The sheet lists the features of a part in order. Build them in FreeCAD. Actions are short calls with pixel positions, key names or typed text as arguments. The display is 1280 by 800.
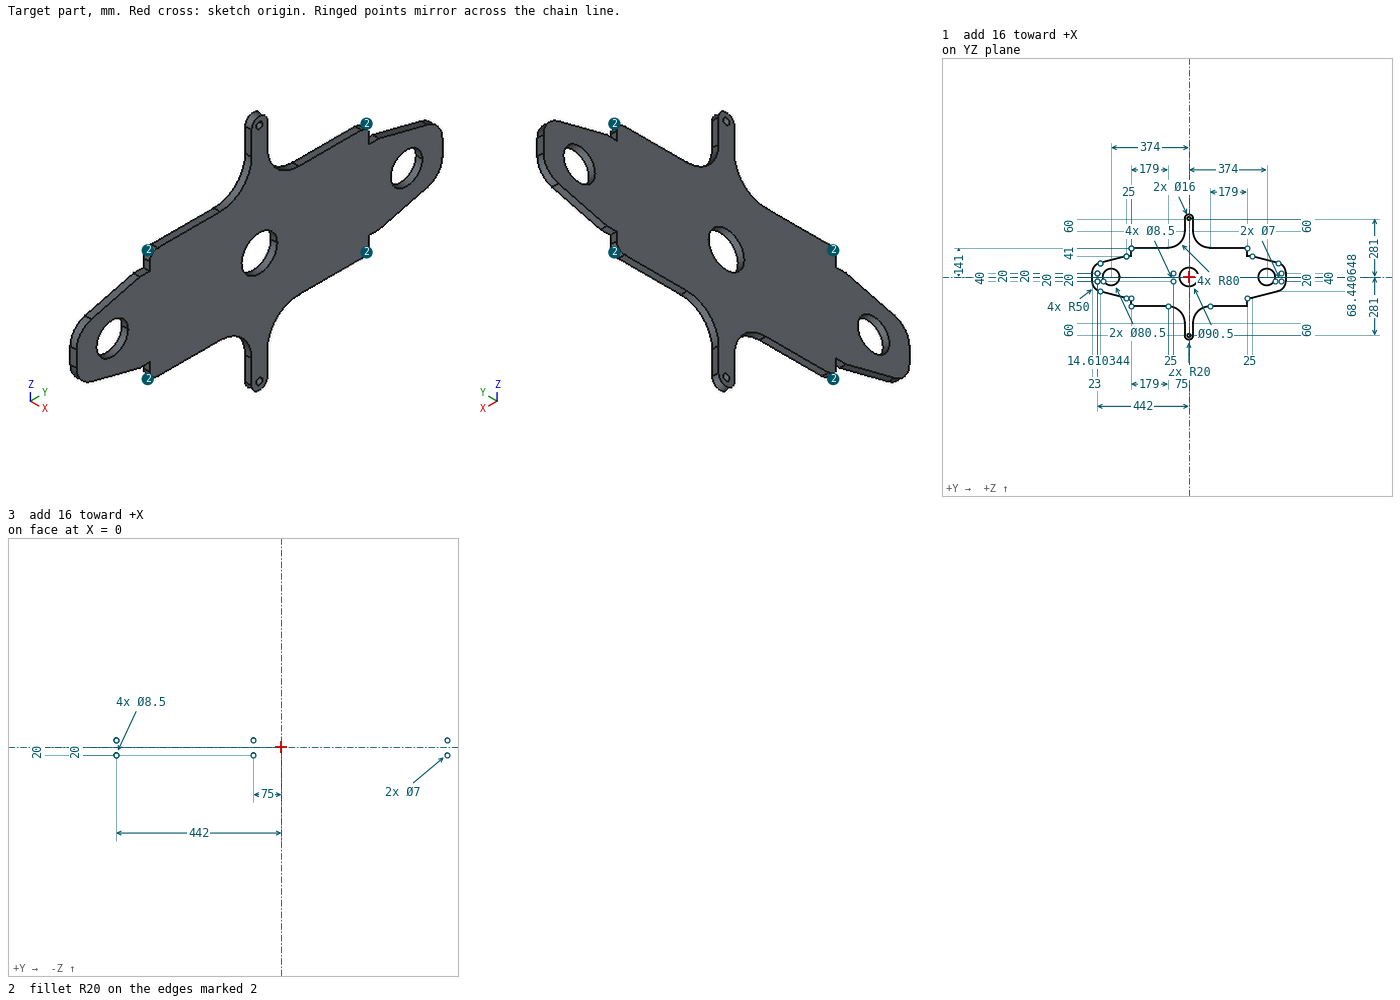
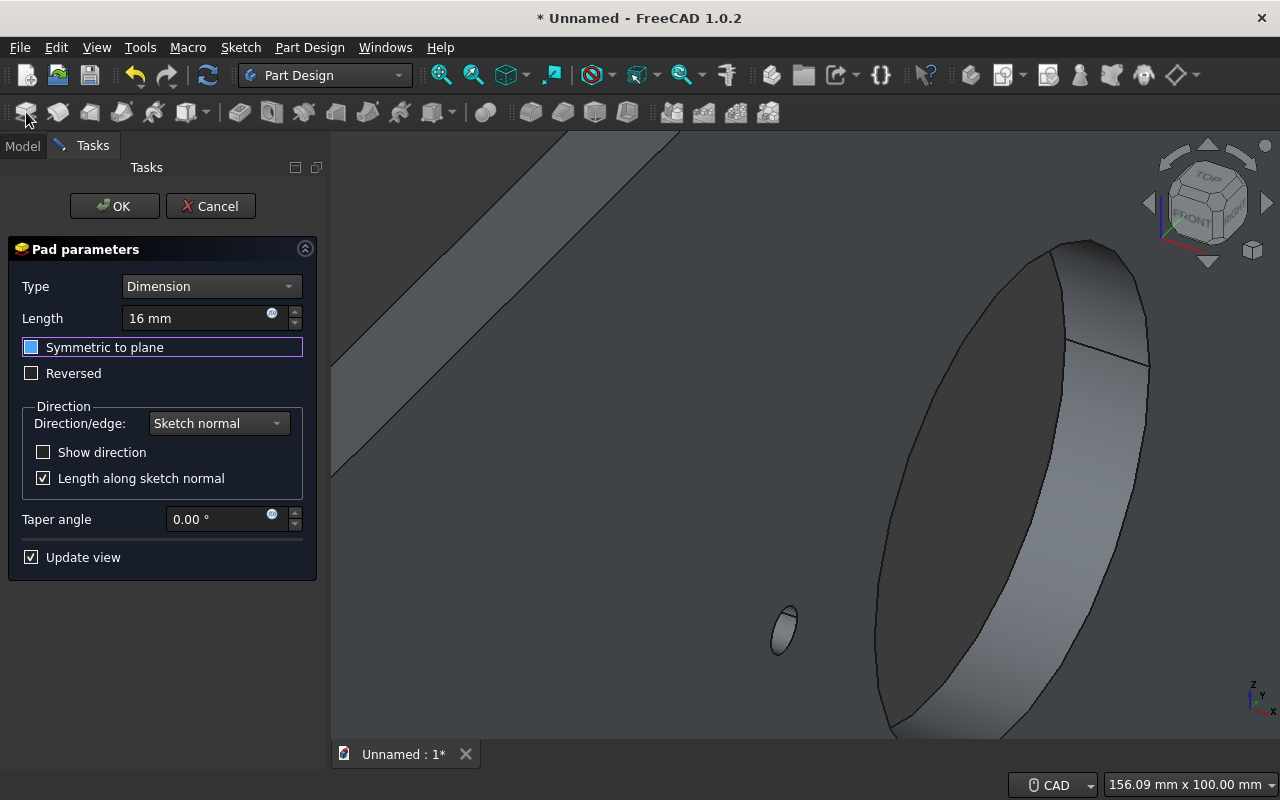
click(115, 206)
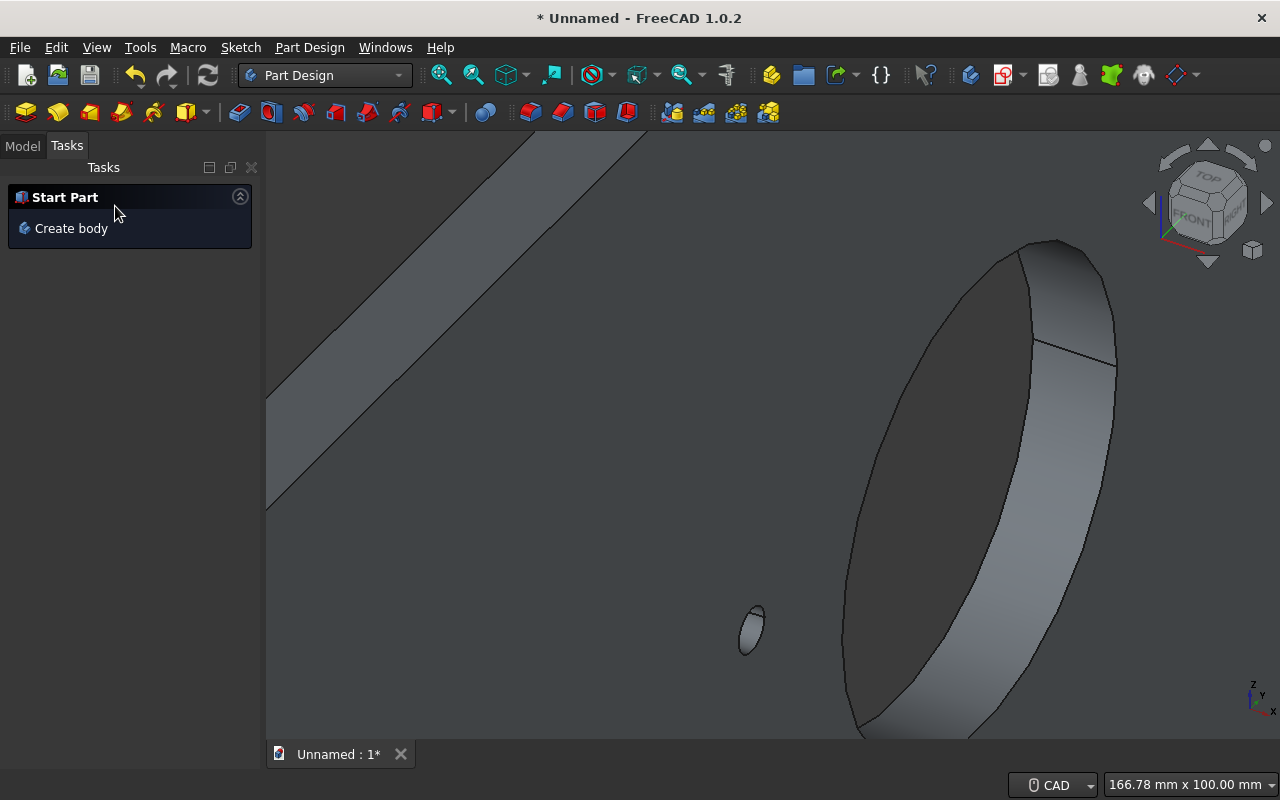
key(v)
key(f)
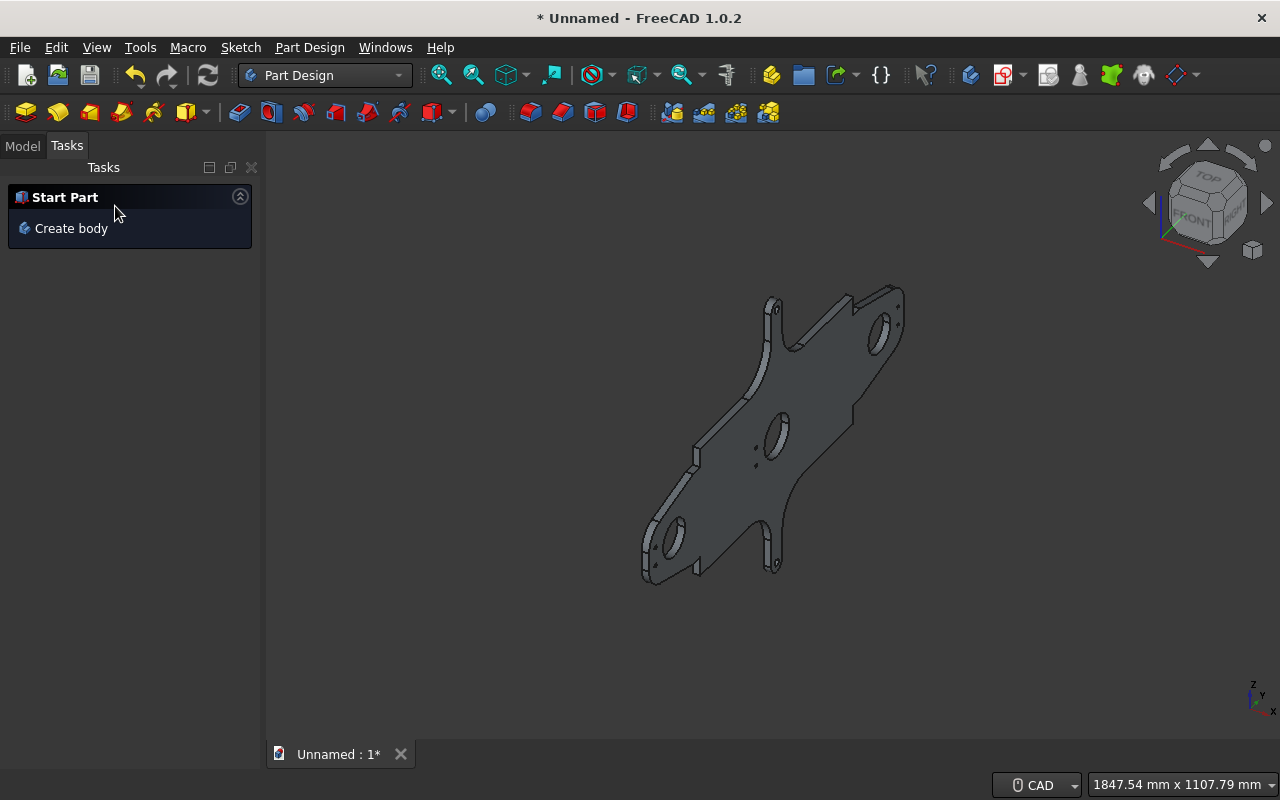
click(694, 446)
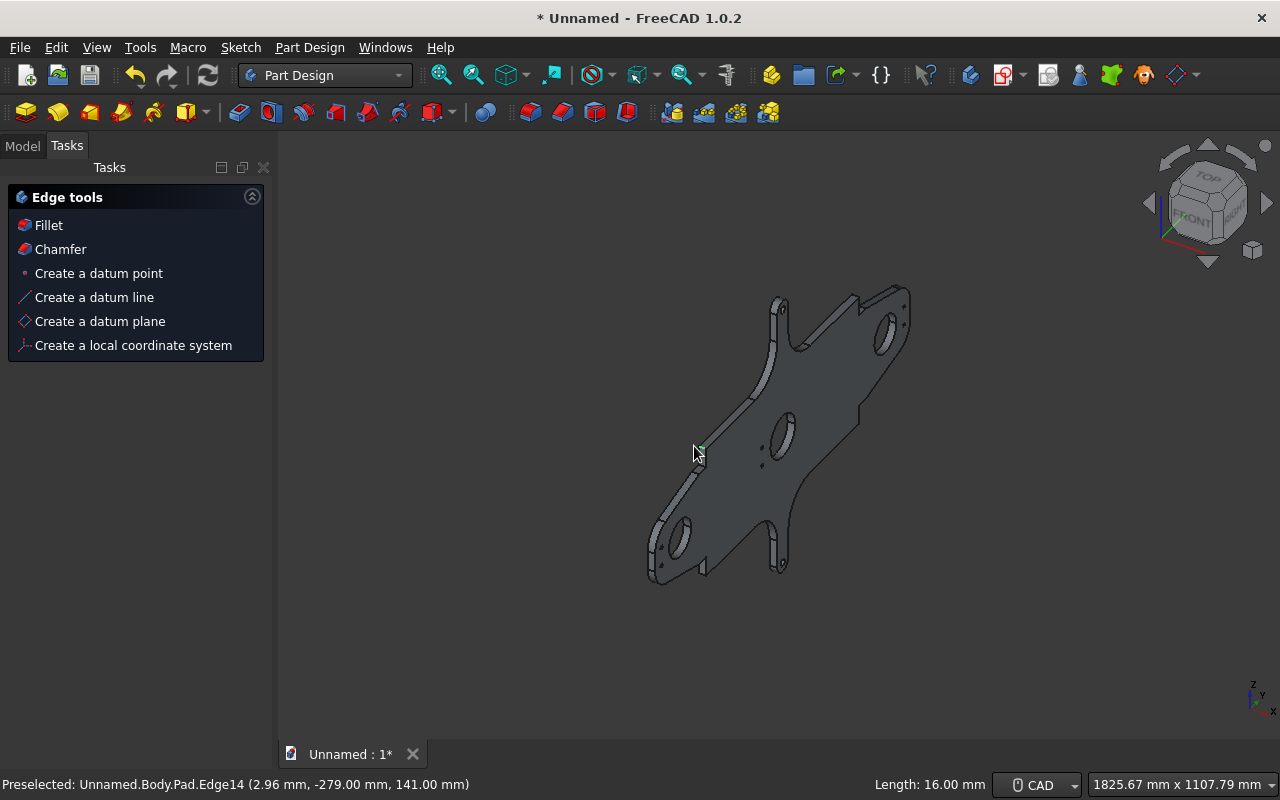
scroll(856, 421, up, 8)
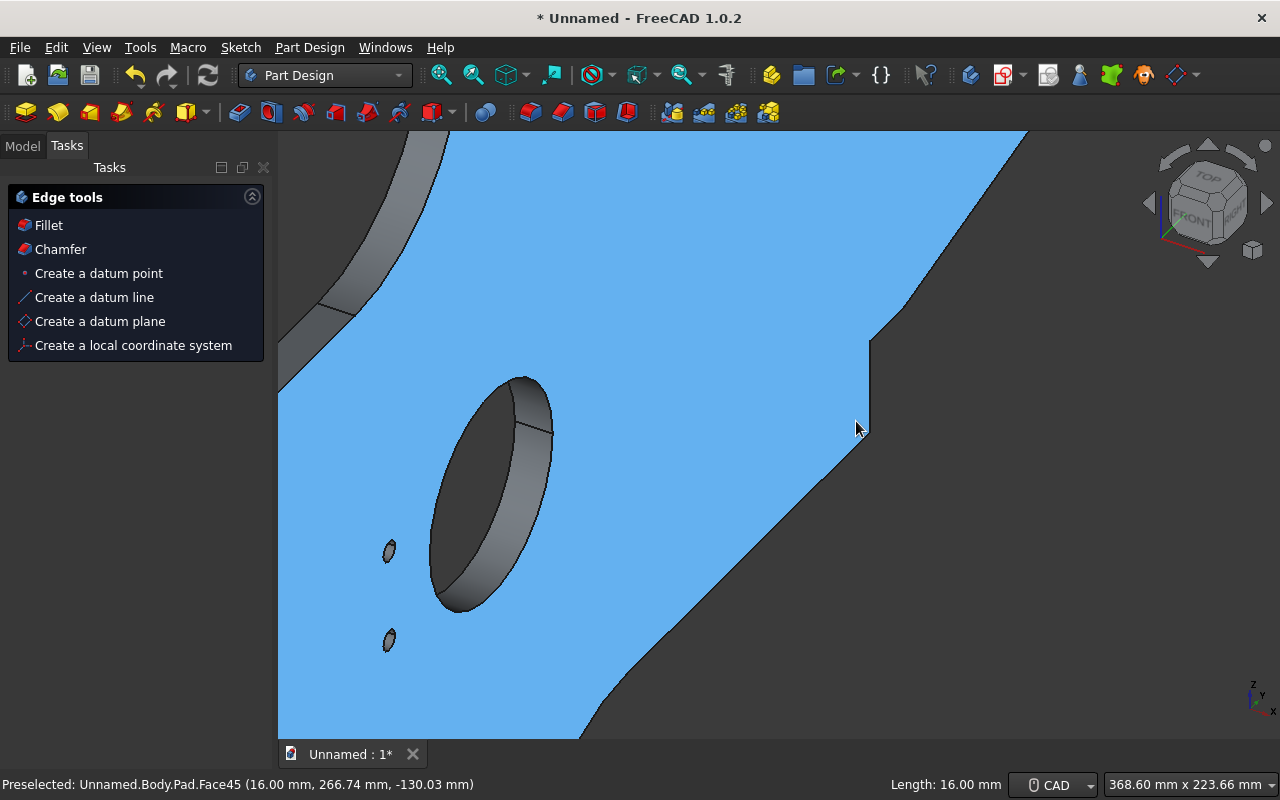
click(442, 76)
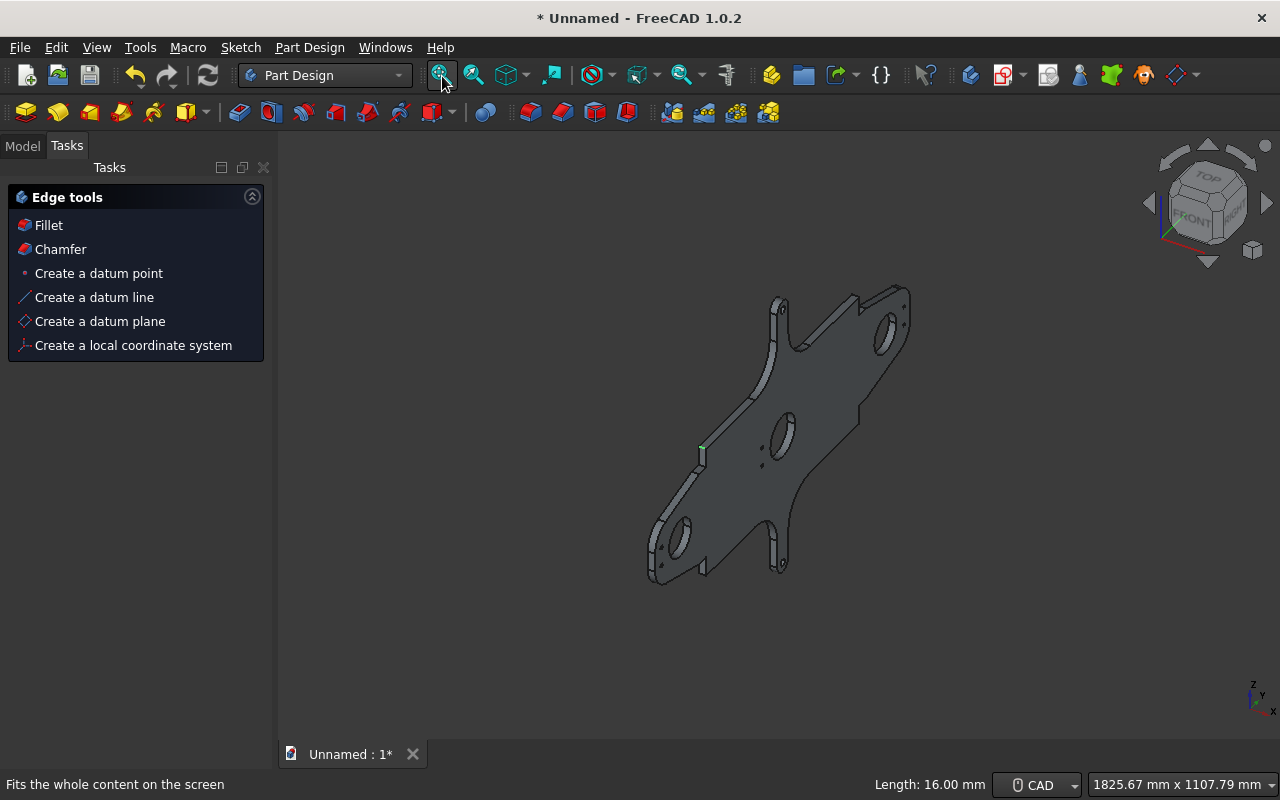
key(0)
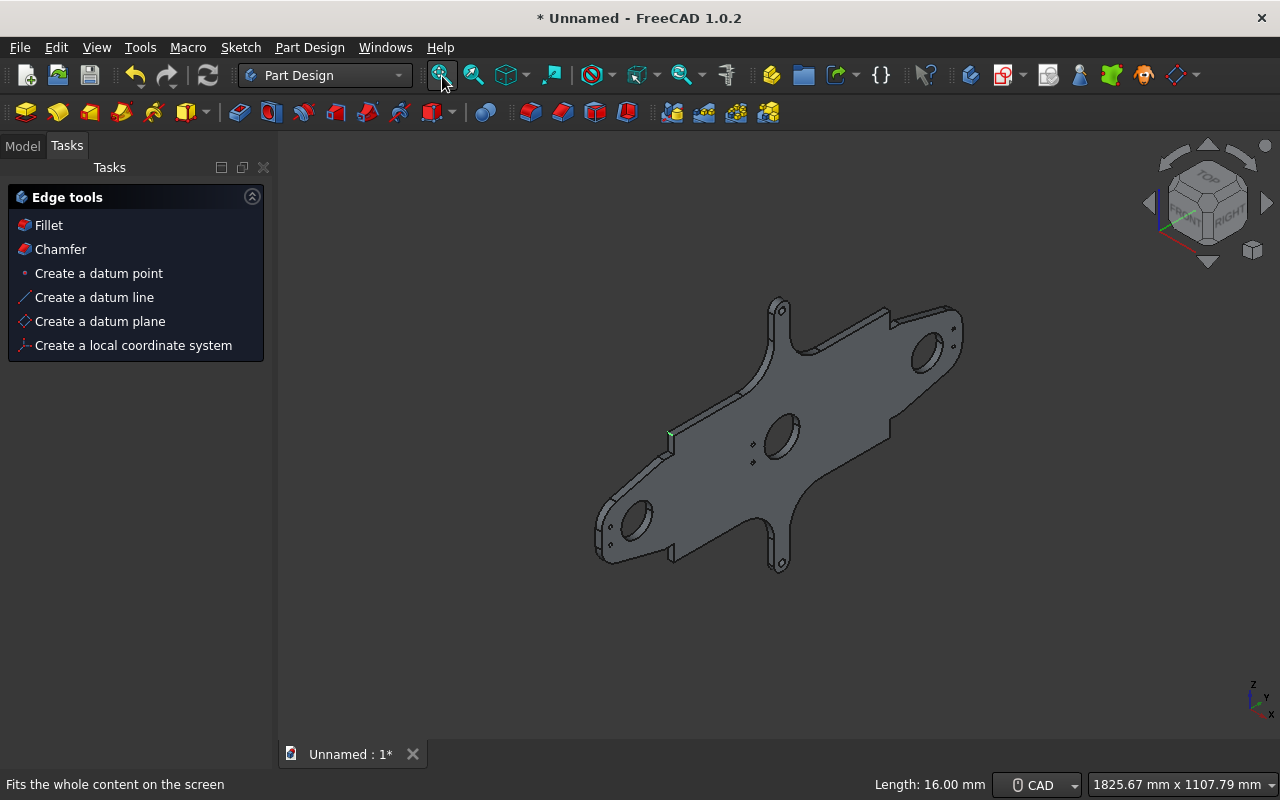
scroll(887, 435, up, 8)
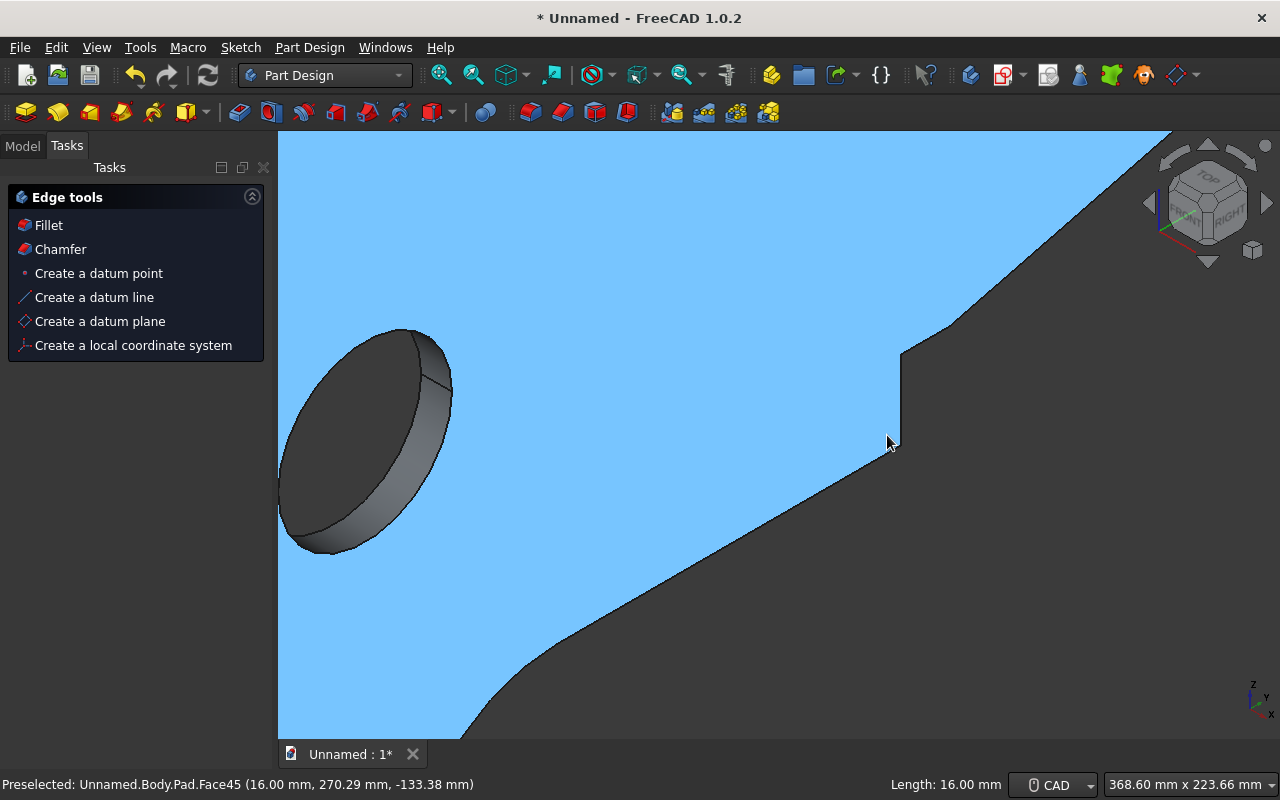
click(442, 76)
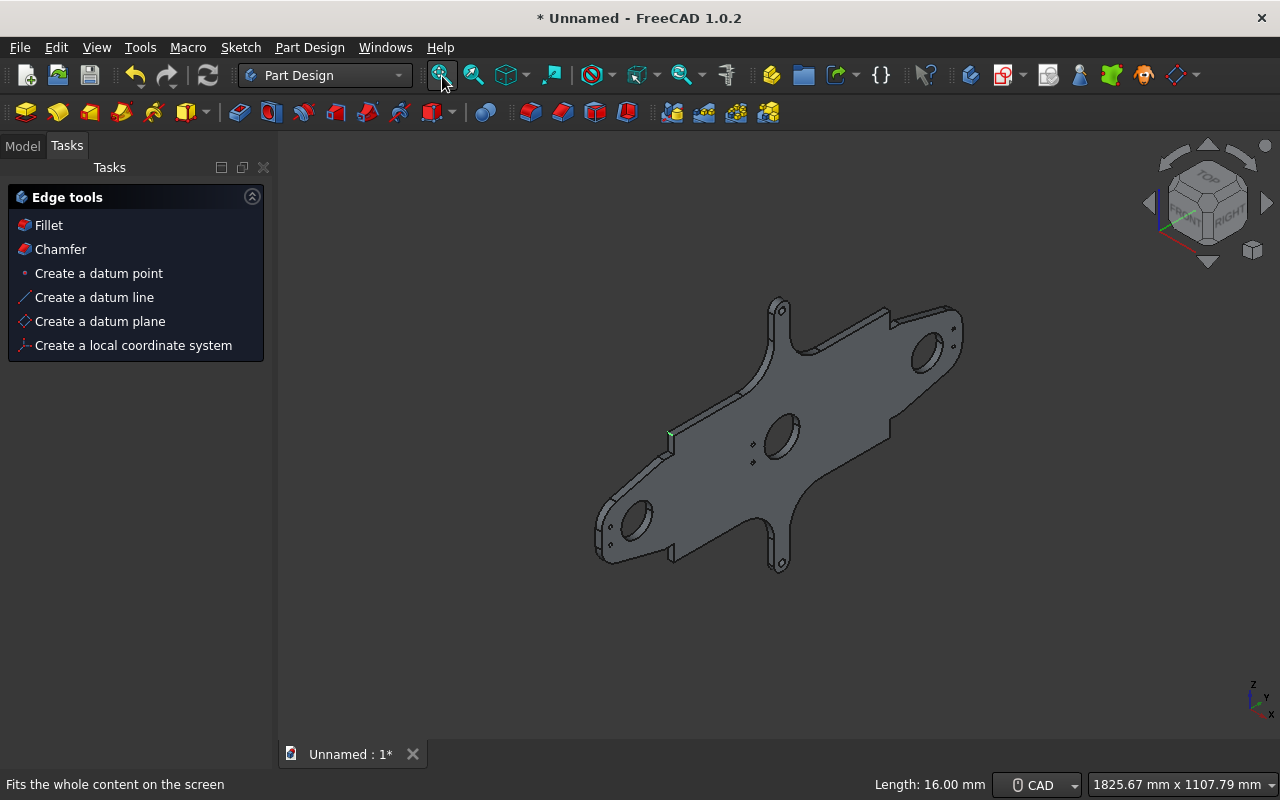
key(2)